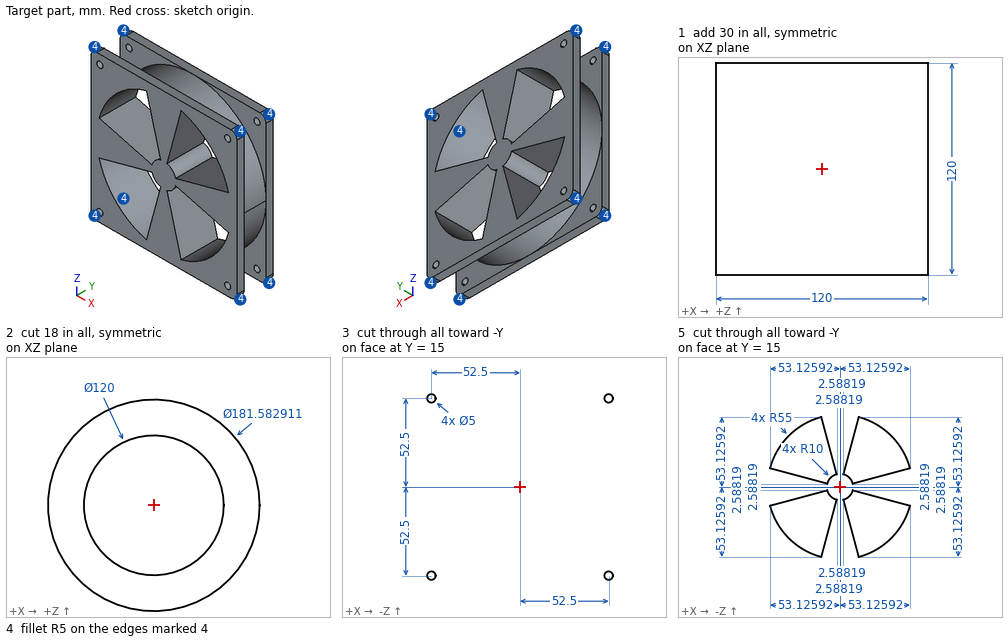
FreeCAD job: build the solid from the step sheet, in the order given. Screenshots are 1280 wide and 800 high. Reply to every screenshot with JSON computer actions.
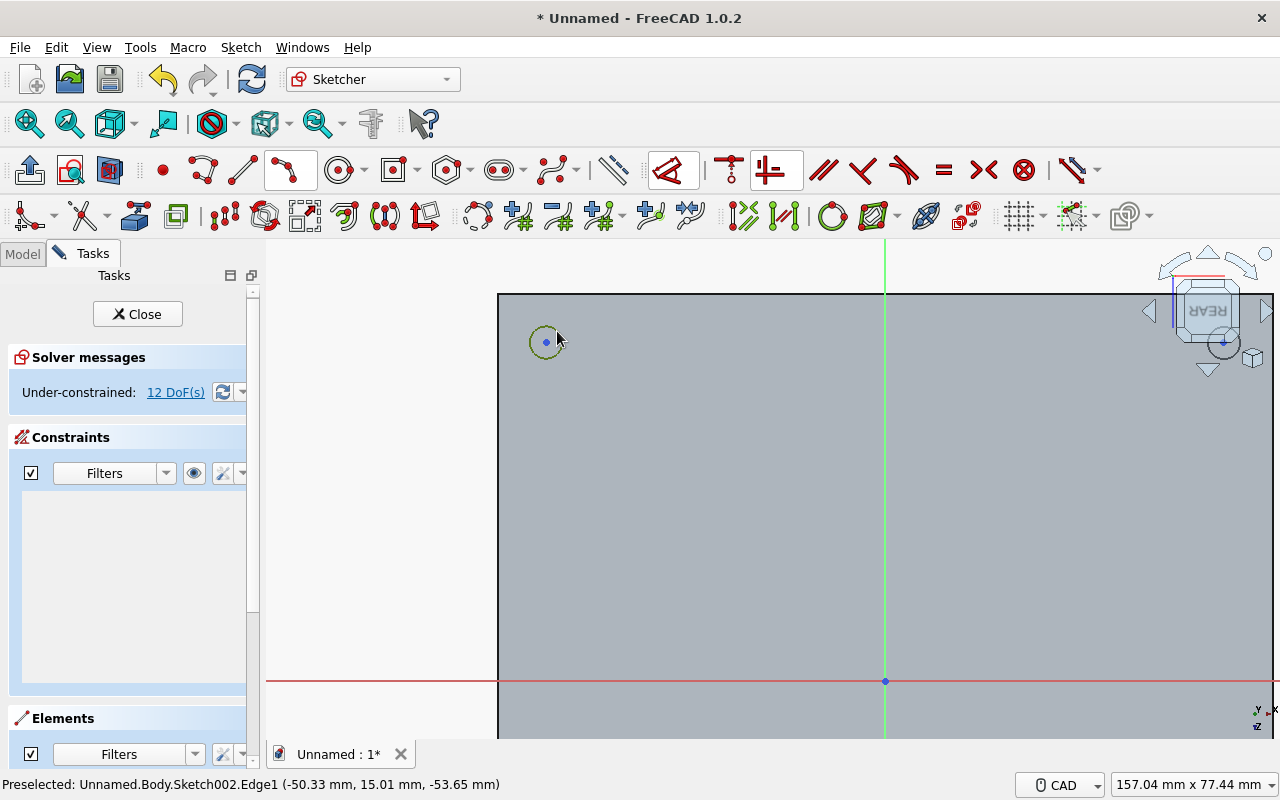
{"action": "scroll", "coordinate": [557, 332], "scroll_direction": "down", "scroll_amount": 4}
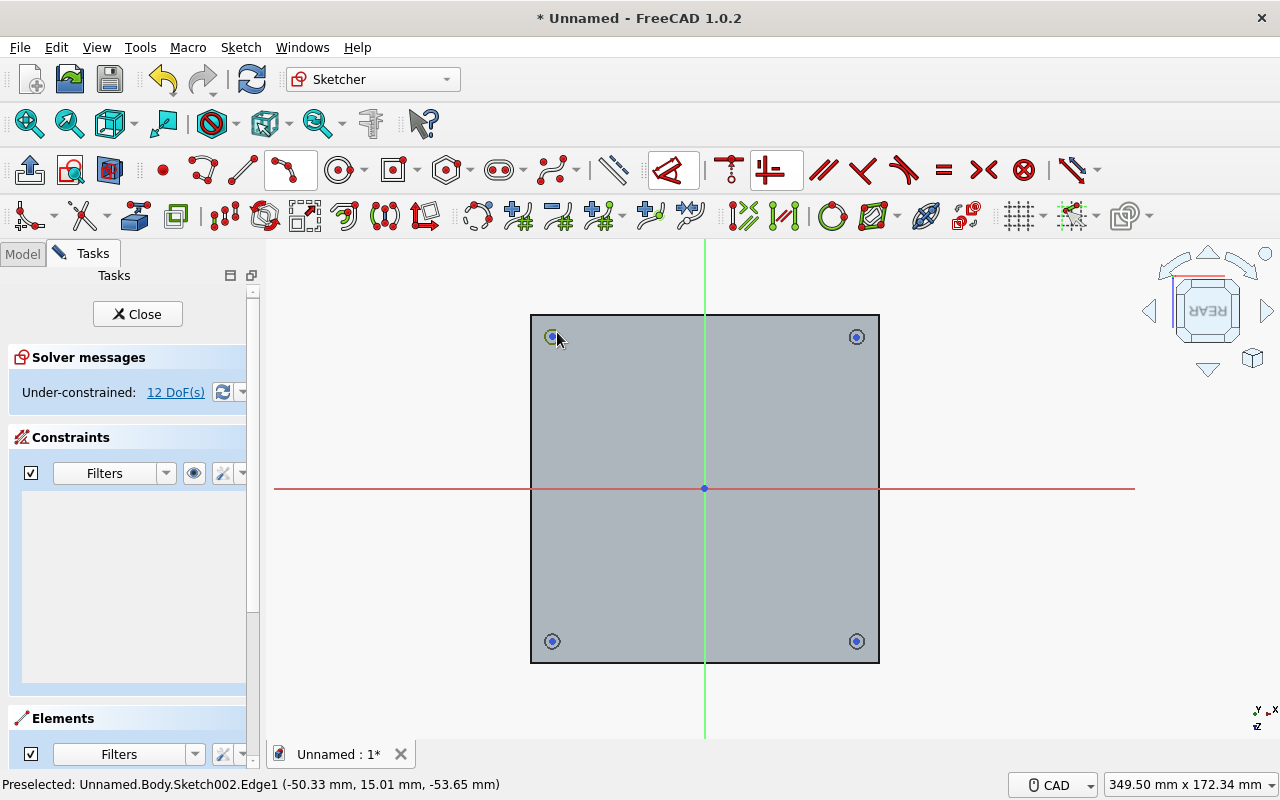
{"action": "scroll", "coordinate": [557, 636], "scroll_direction": "up", "scroll_amount": 4}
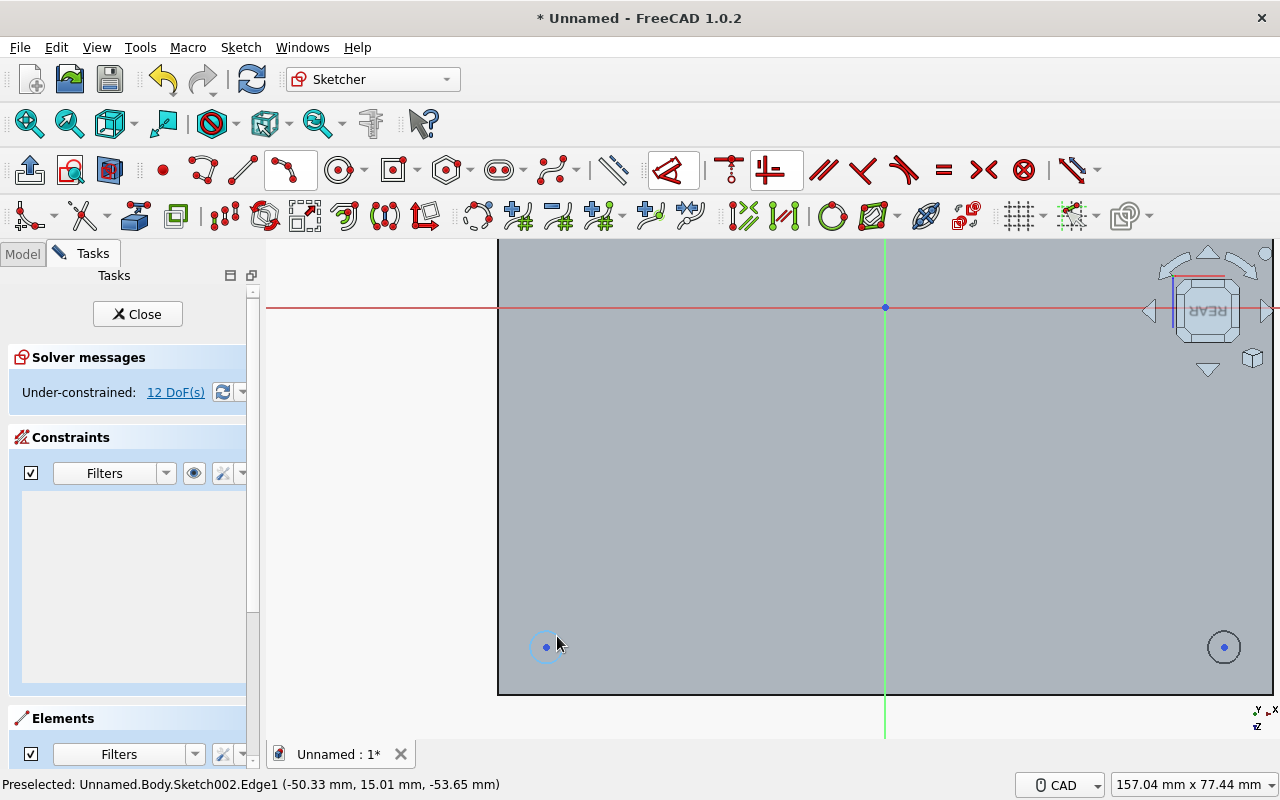
{"action": "left_click", "coordinate": [558, 636]}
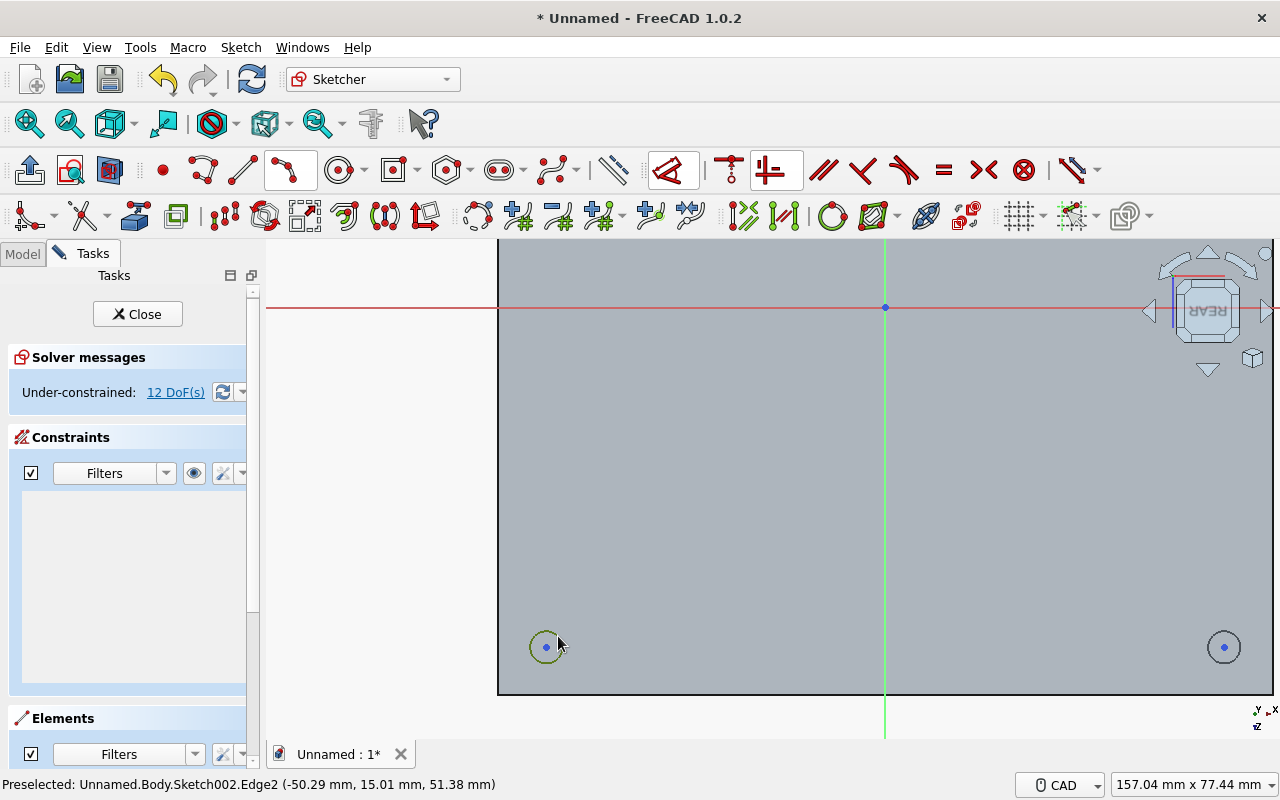
{"action": "scroll", "coordinate": [557, 637], "scroll_direction": "down", "scroll_amount": 4}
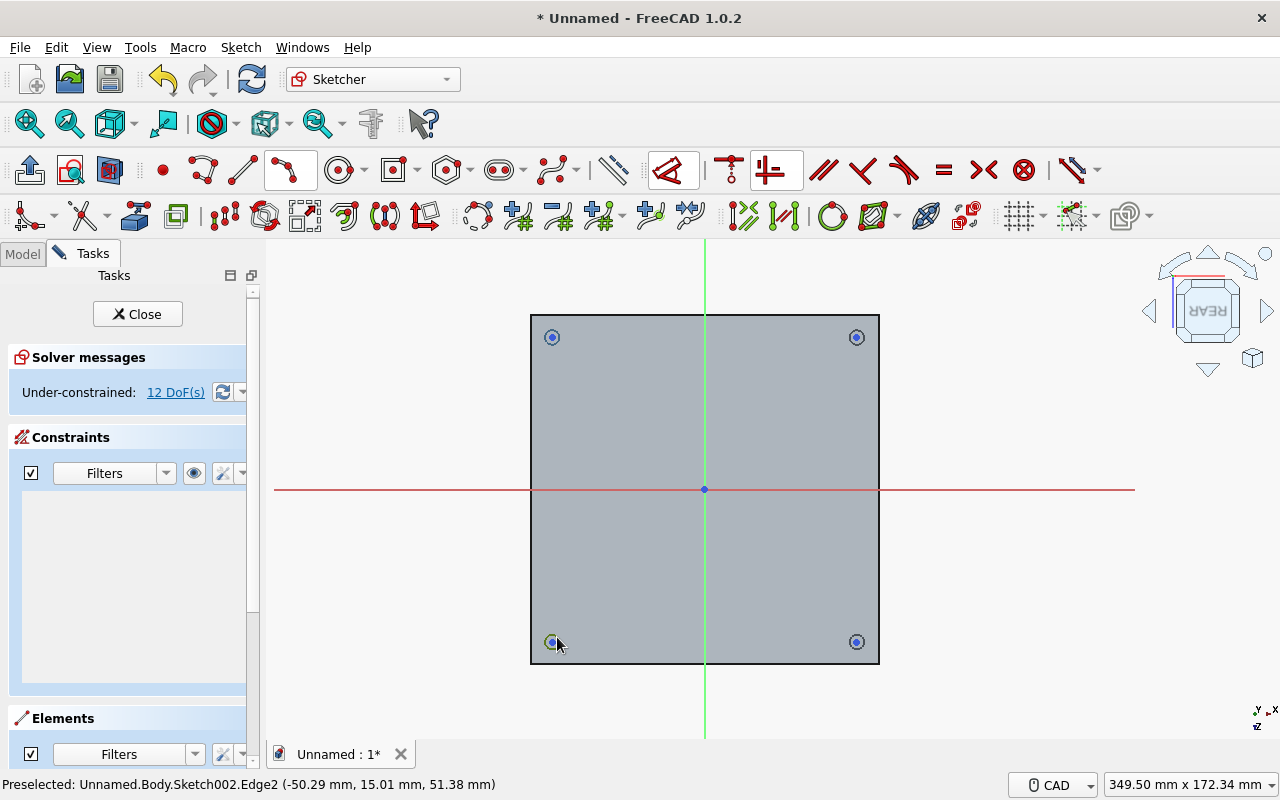
{"action": "scroll", "coordinate": [862, 637], "scroll_direction": "up", "scroll_amount": 4}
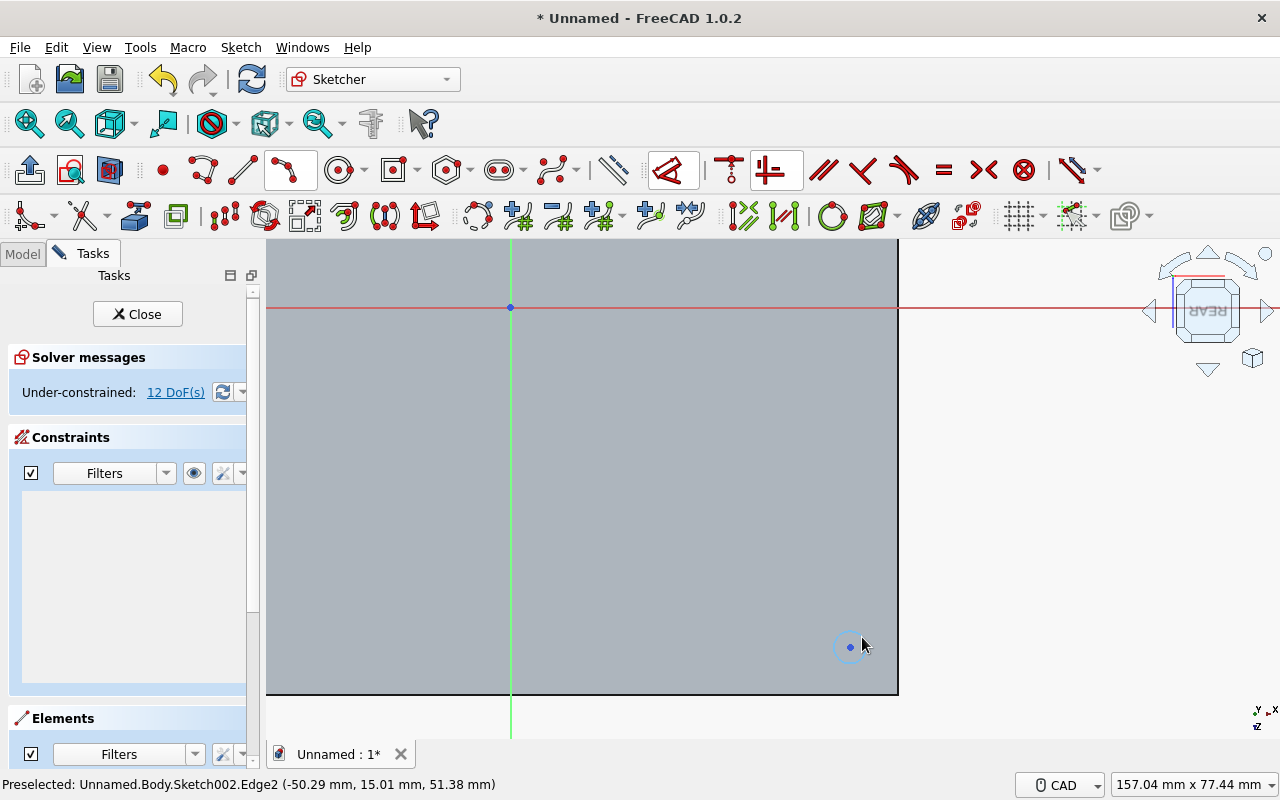
{"action": "left_click", "coordinate": [861, 636]}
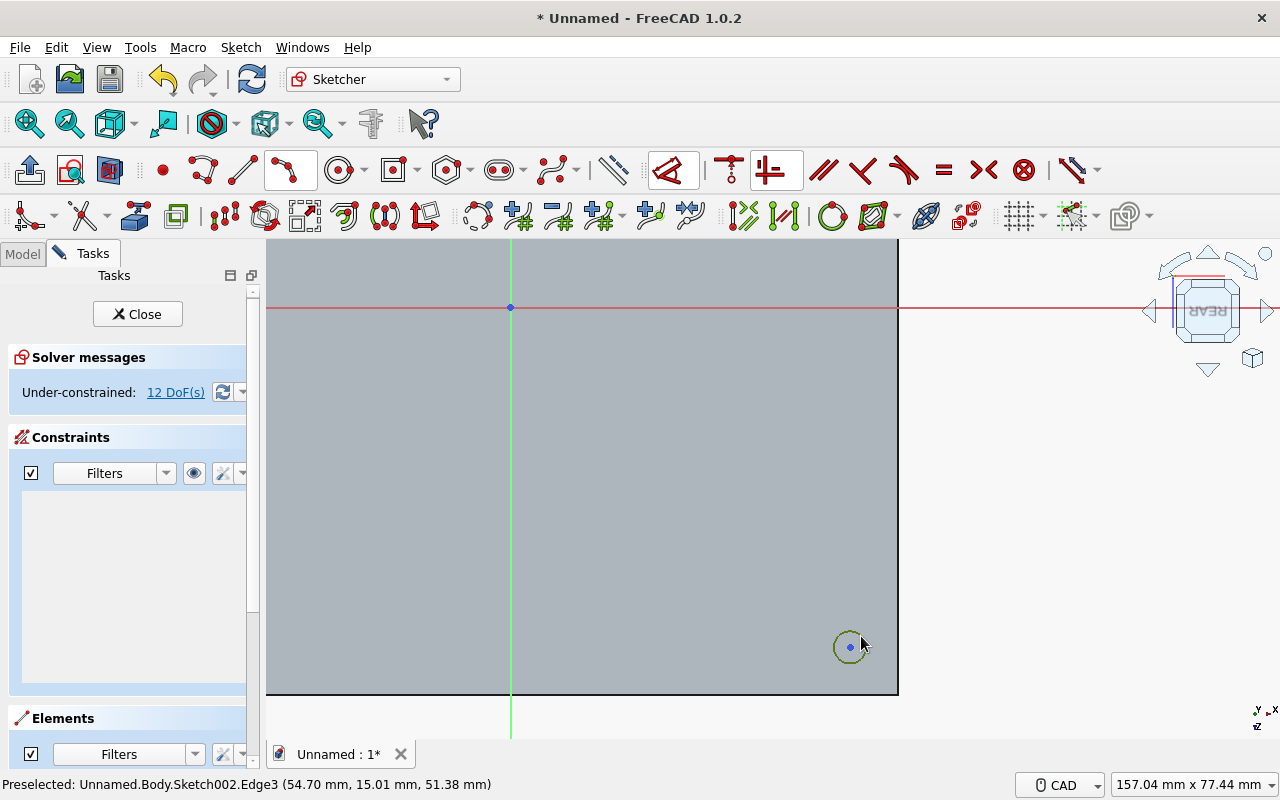
{"action": "scroll", "coordinate": [862, 637], "scroll_direction": "down", "scroll_amount": 4}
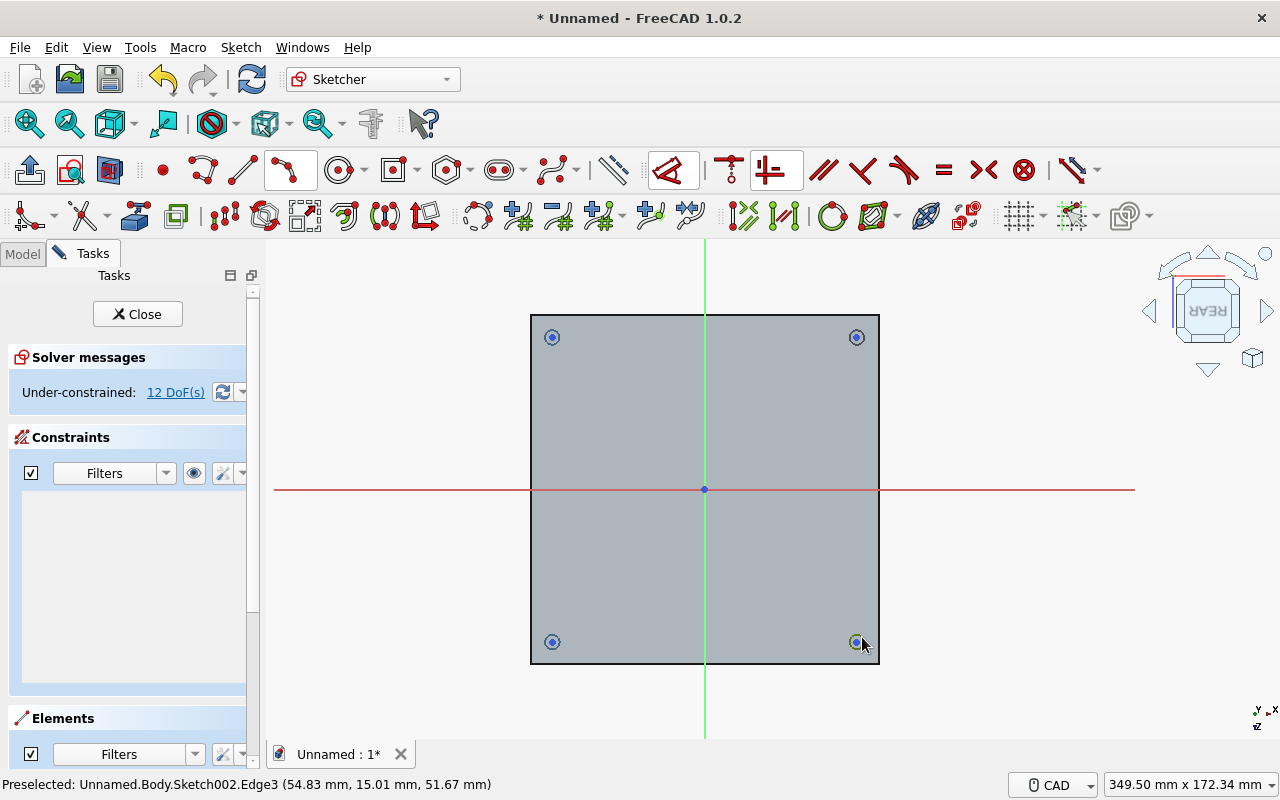
{"action": "scroll", "coordinate": [862, 332], "scroll_direction": "up", "scroll_amount": 4}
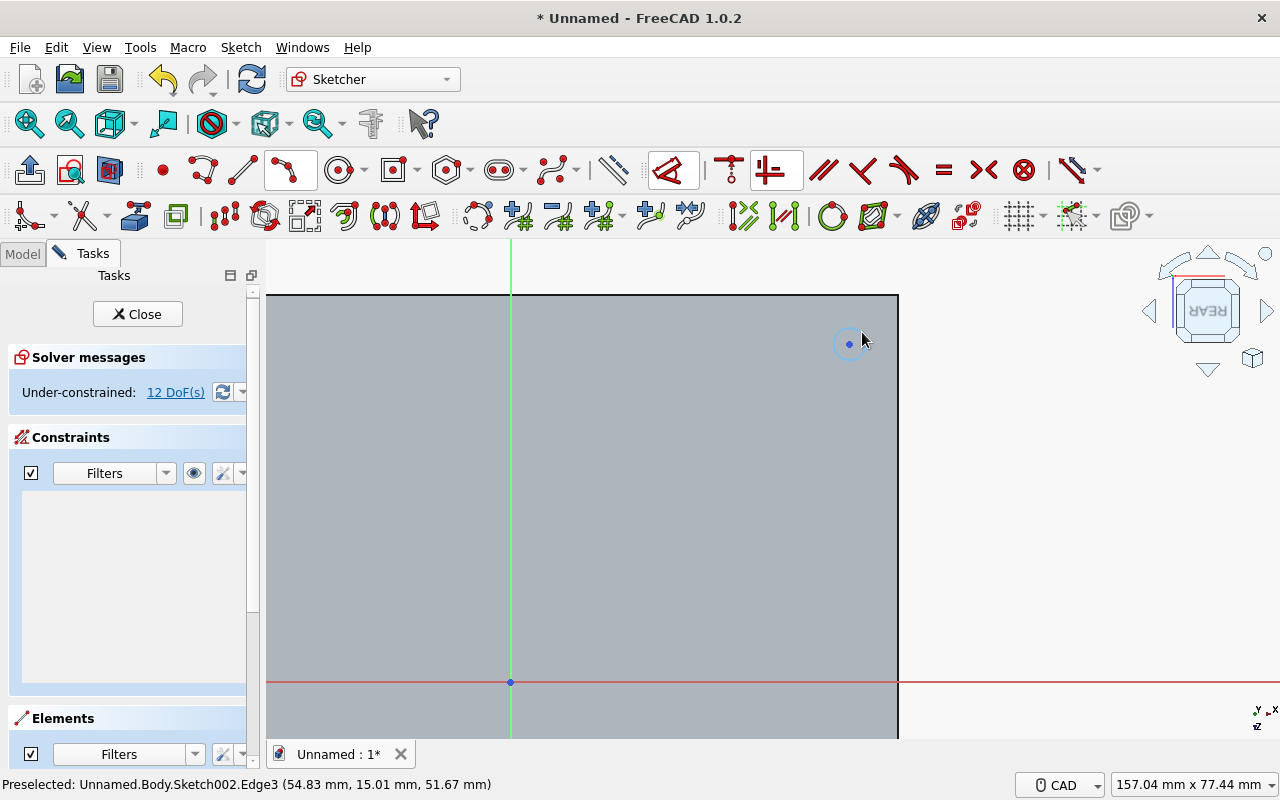
{"action": "left_click", "coordinate": [861, 333]}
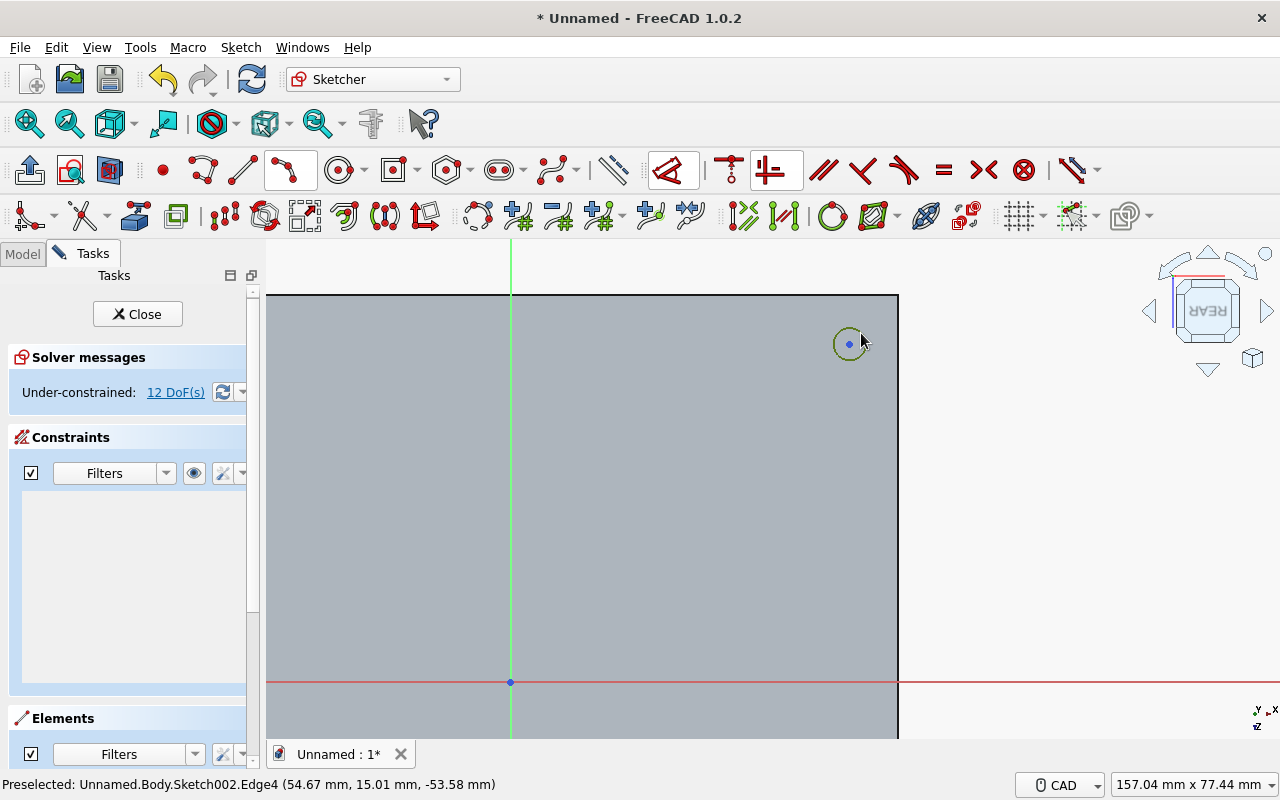
{"action": "left_click", "coordinate": [944, 170]}